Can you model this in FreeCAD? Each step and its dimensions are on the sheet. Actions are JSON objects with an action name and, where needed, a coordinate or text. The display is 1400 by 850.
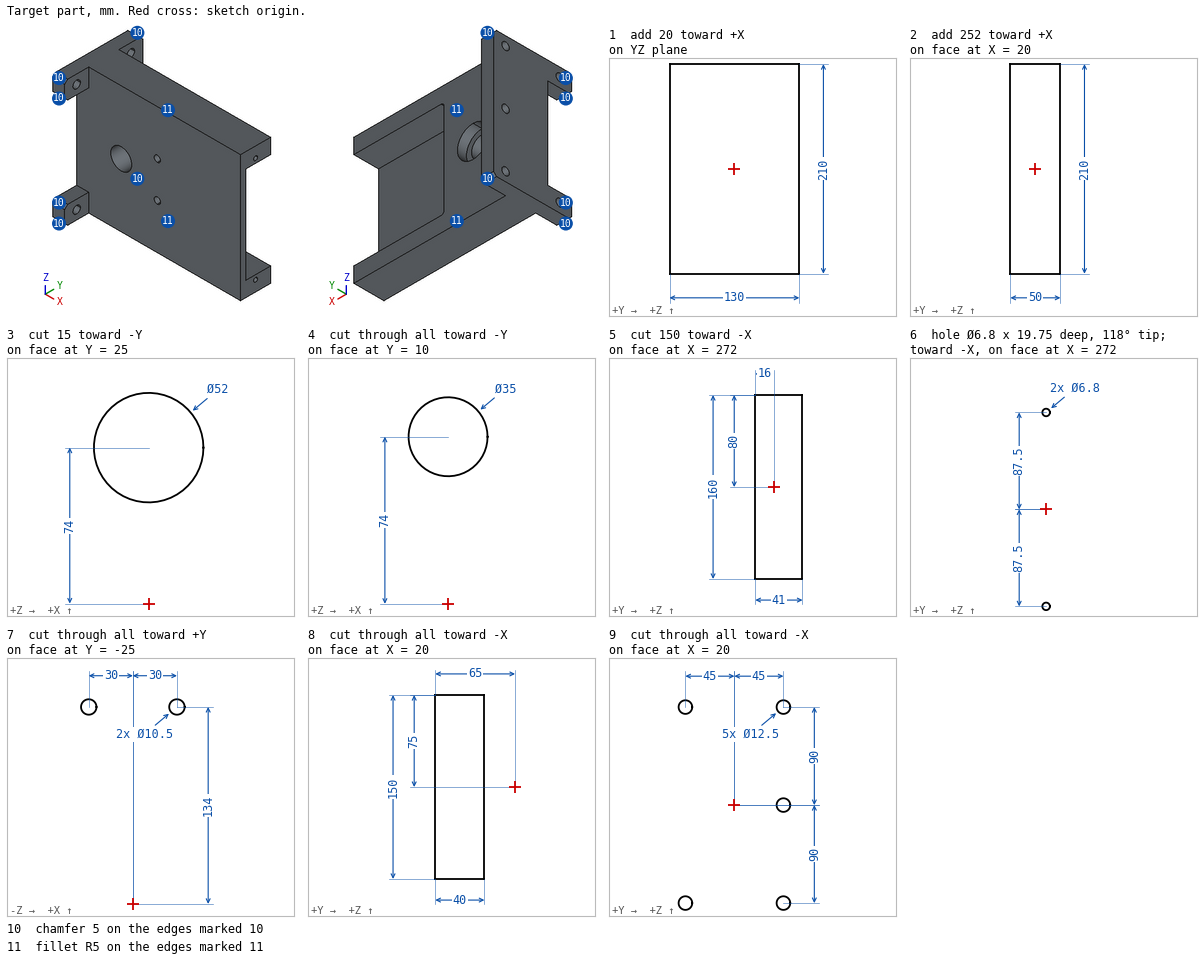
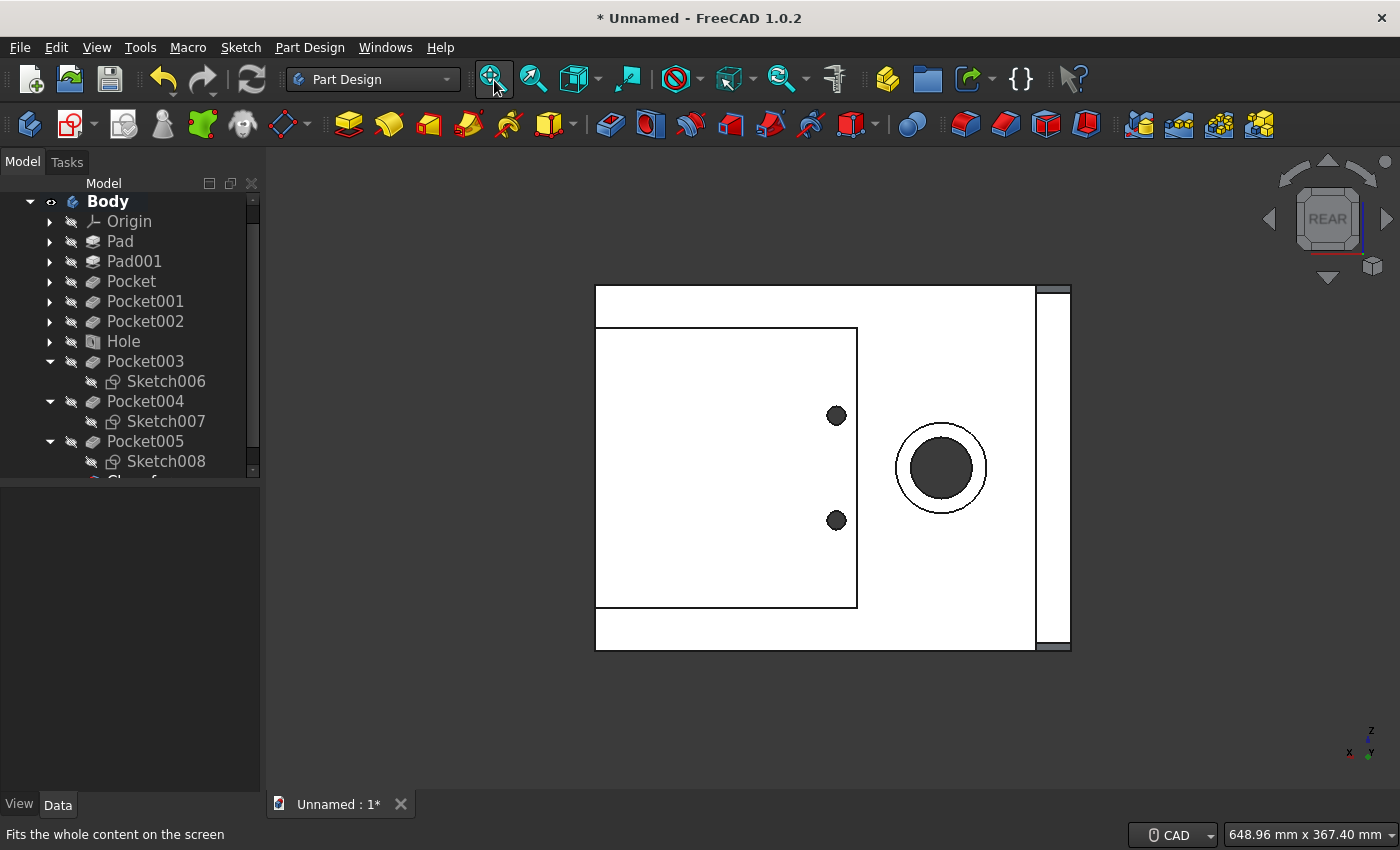
{"action": "key", "text": "6"}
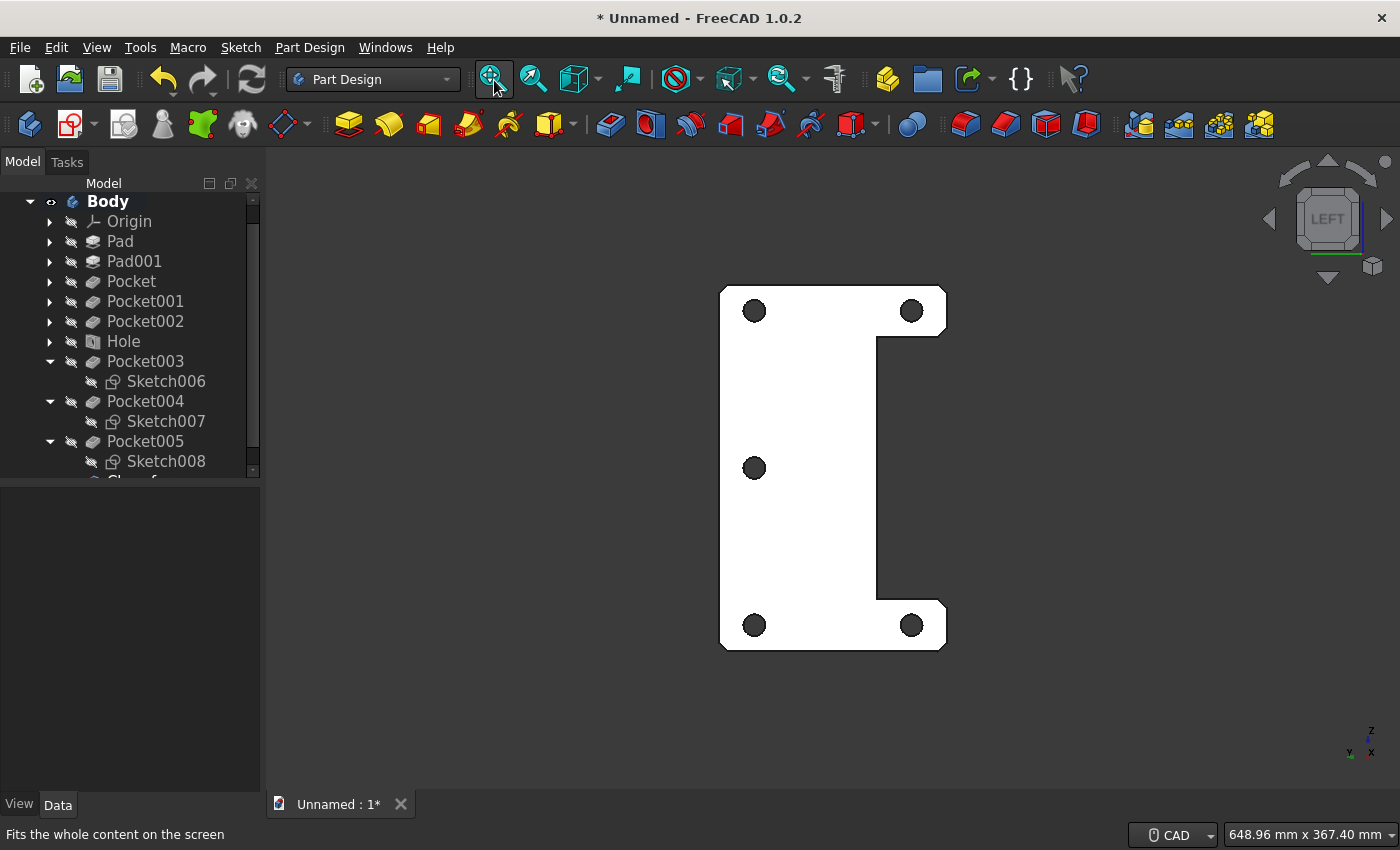
{"action": "key", "text": "v 3"}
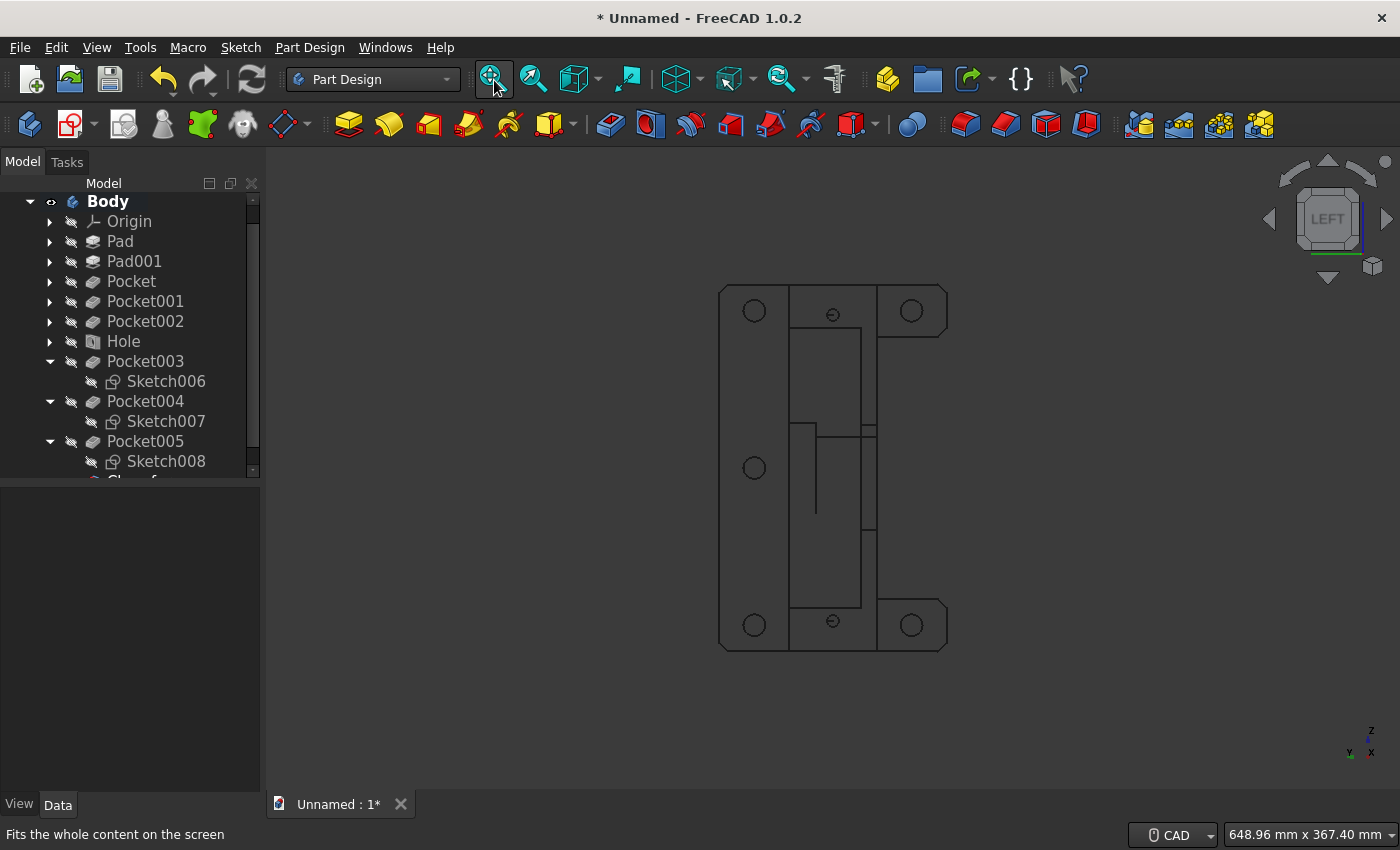
{"action": "key", "text": "0"}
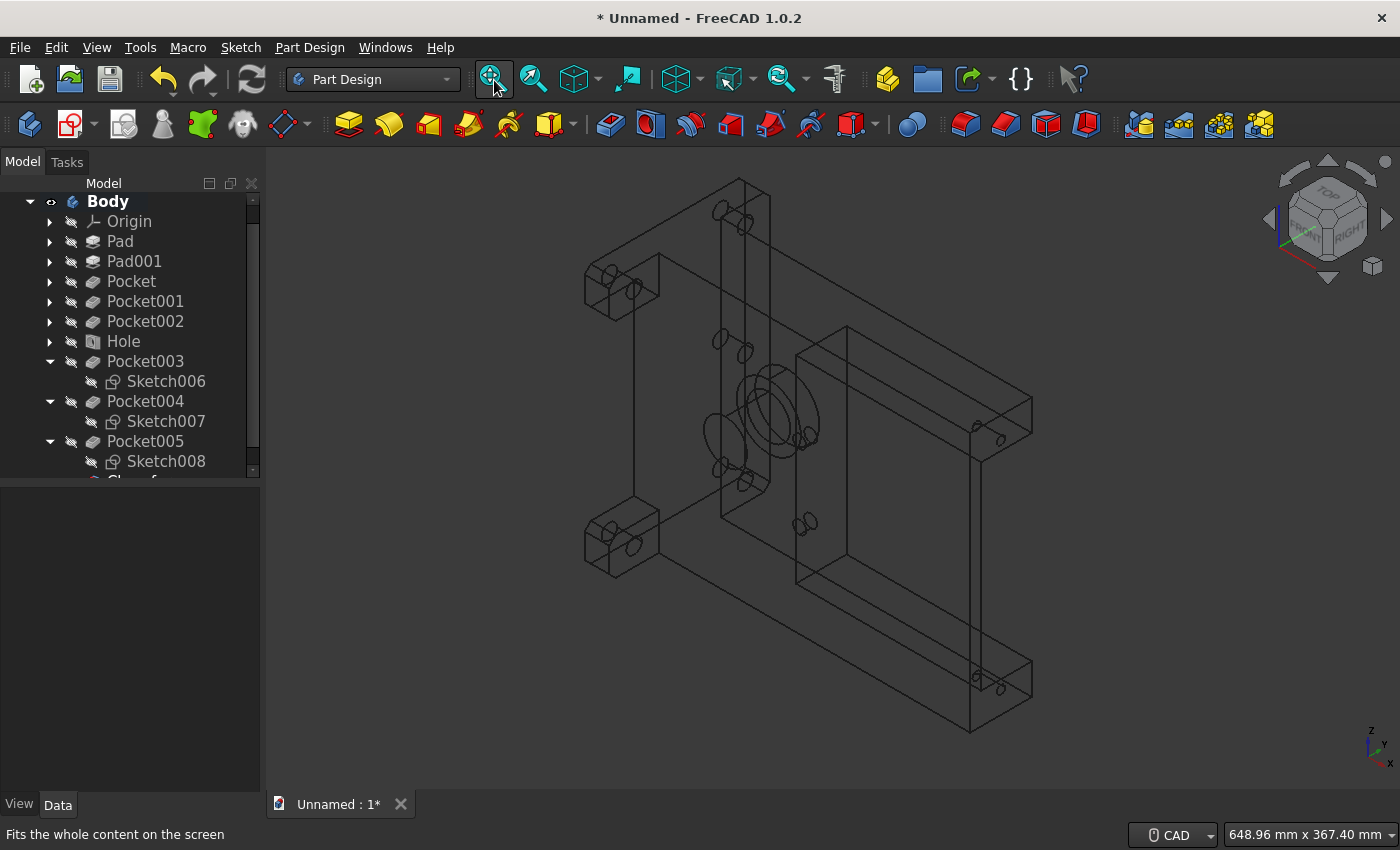
{"action": "left_click", "coordinate": [826, 337]}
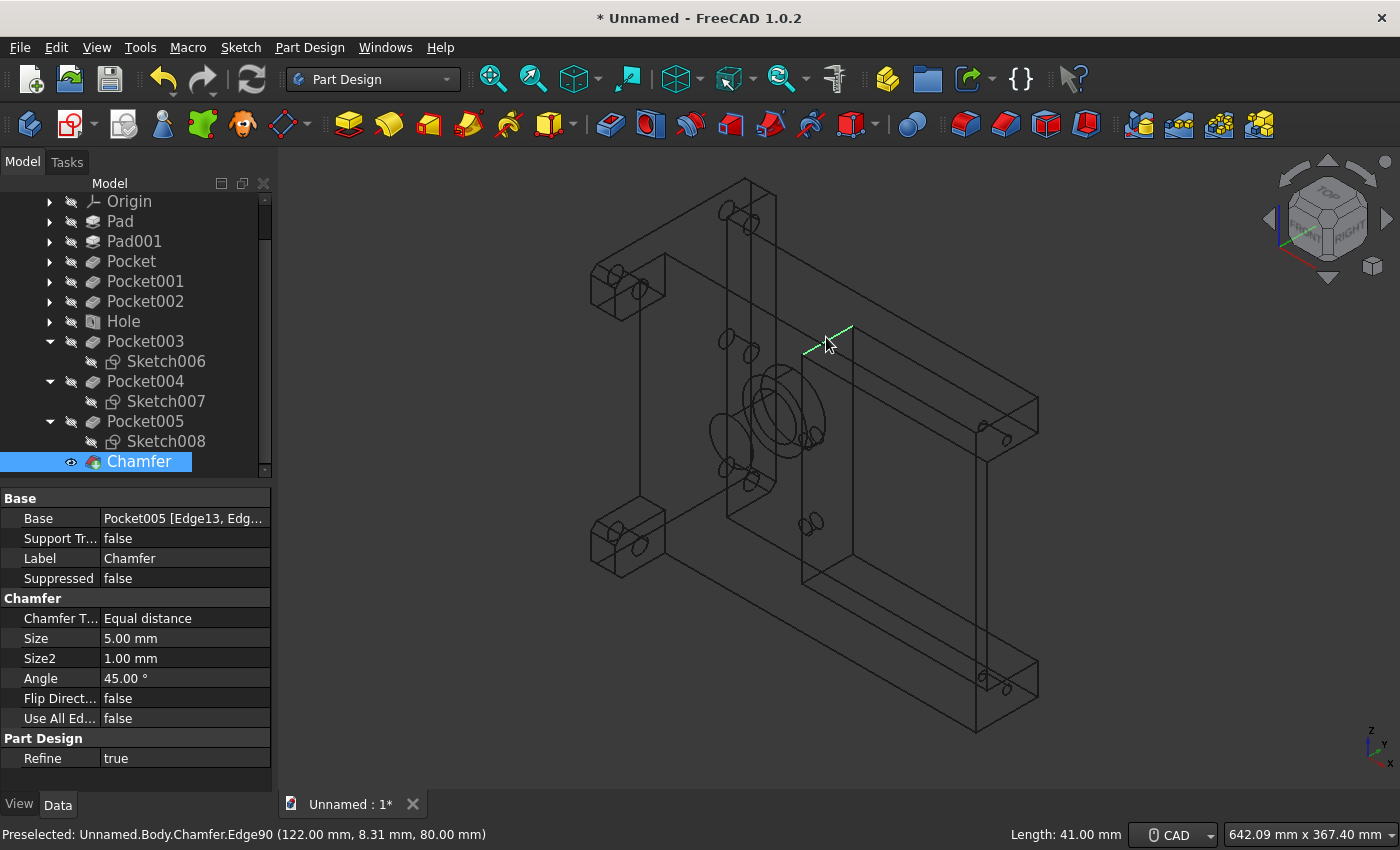
{"action": "left_click", "coordinate": [827, 568], "text": "ctrl"}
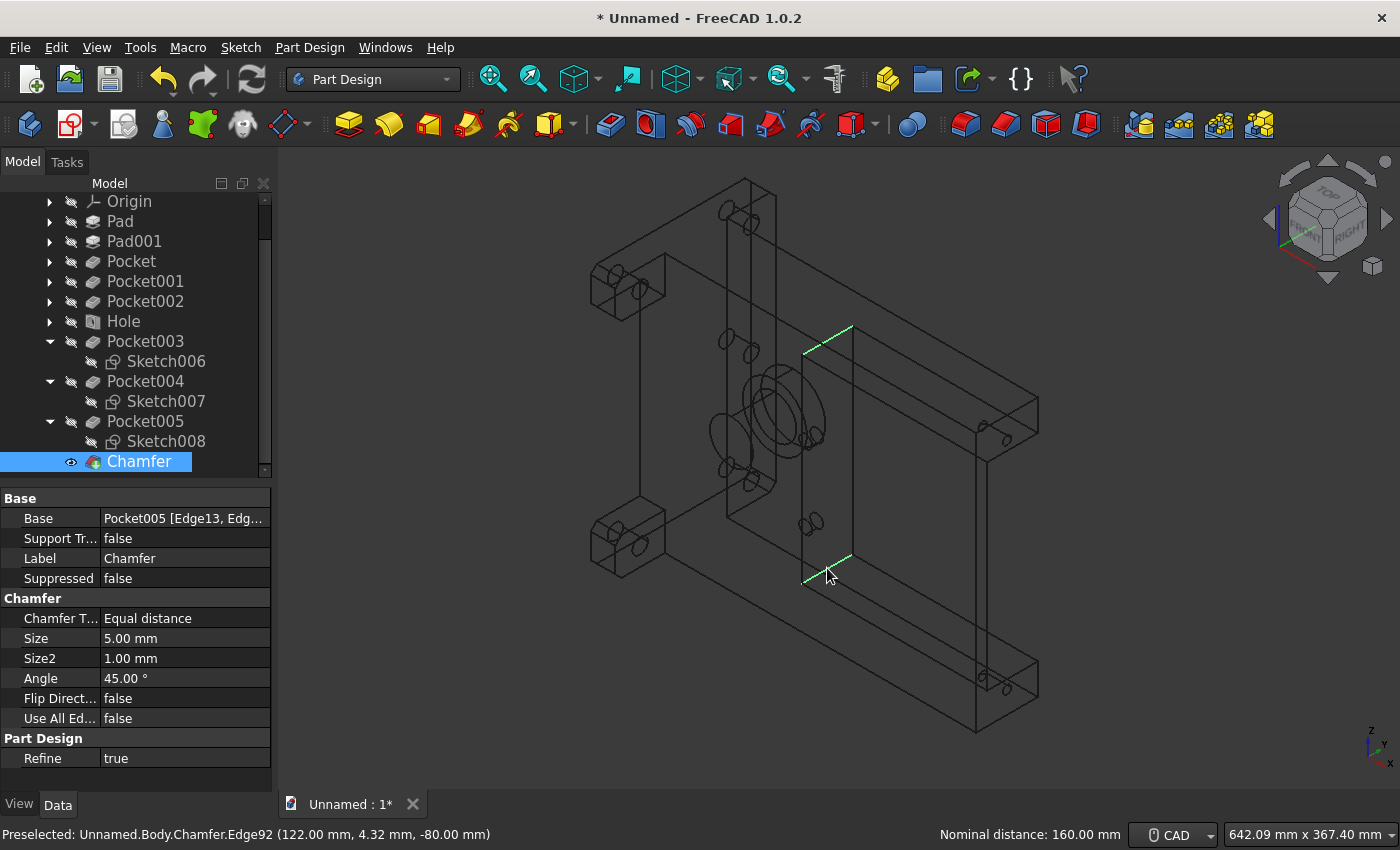
{"action": "key", "text": "v 1"}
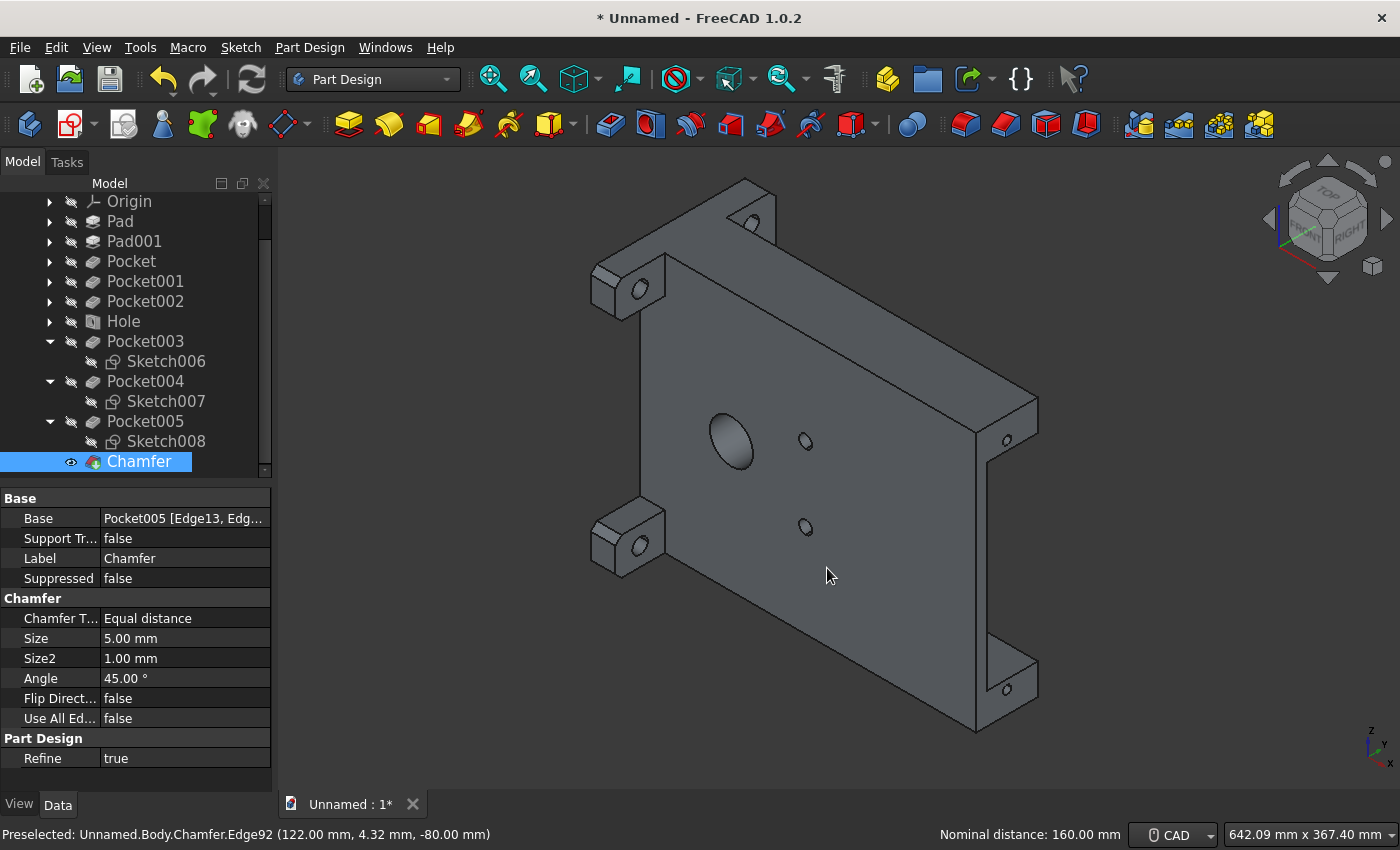
{"action": "left_click", "coordinate": [966, 124]}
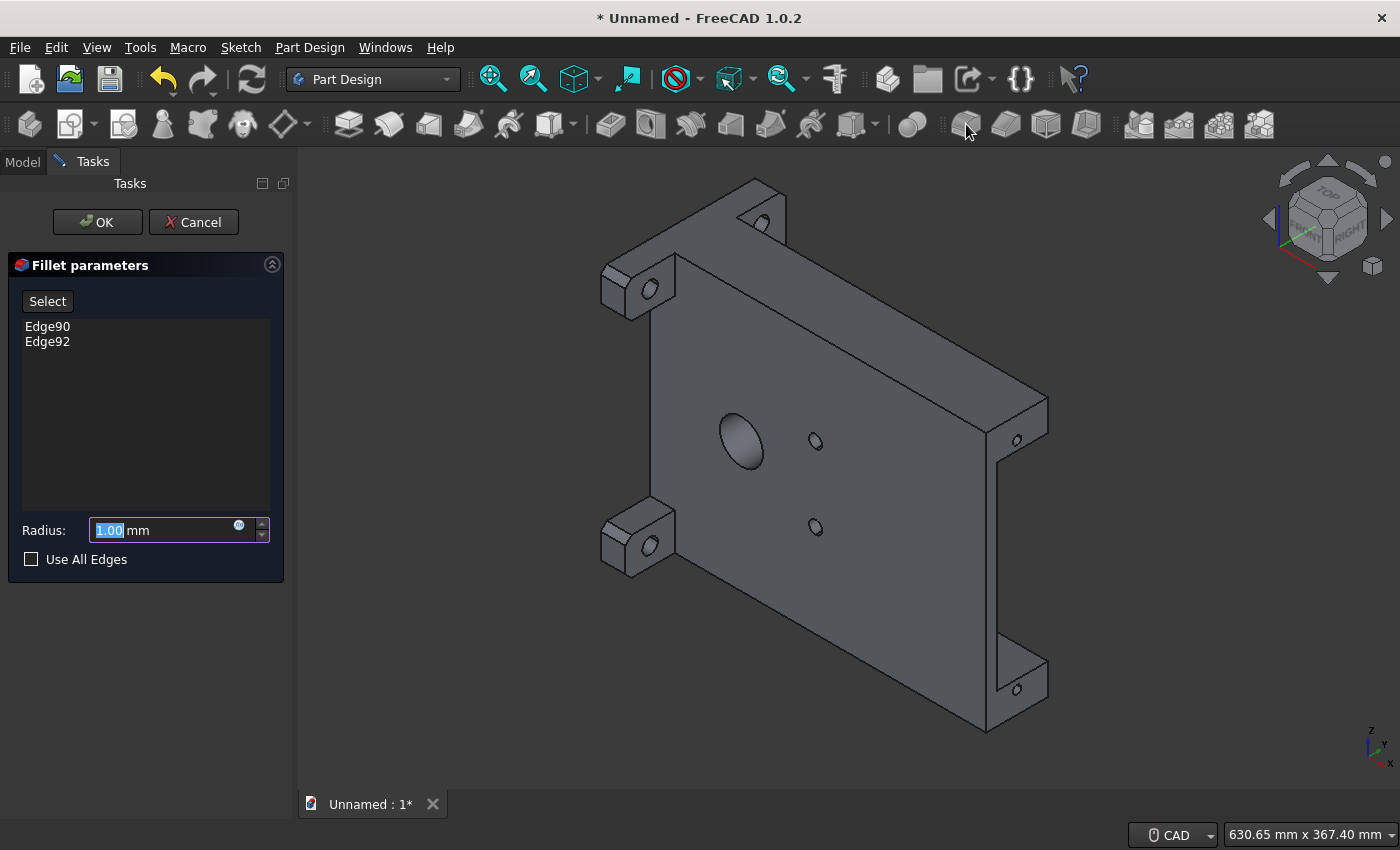
{"action": "type", "text": "5"}
{"action": "key", "text": "Tab"}